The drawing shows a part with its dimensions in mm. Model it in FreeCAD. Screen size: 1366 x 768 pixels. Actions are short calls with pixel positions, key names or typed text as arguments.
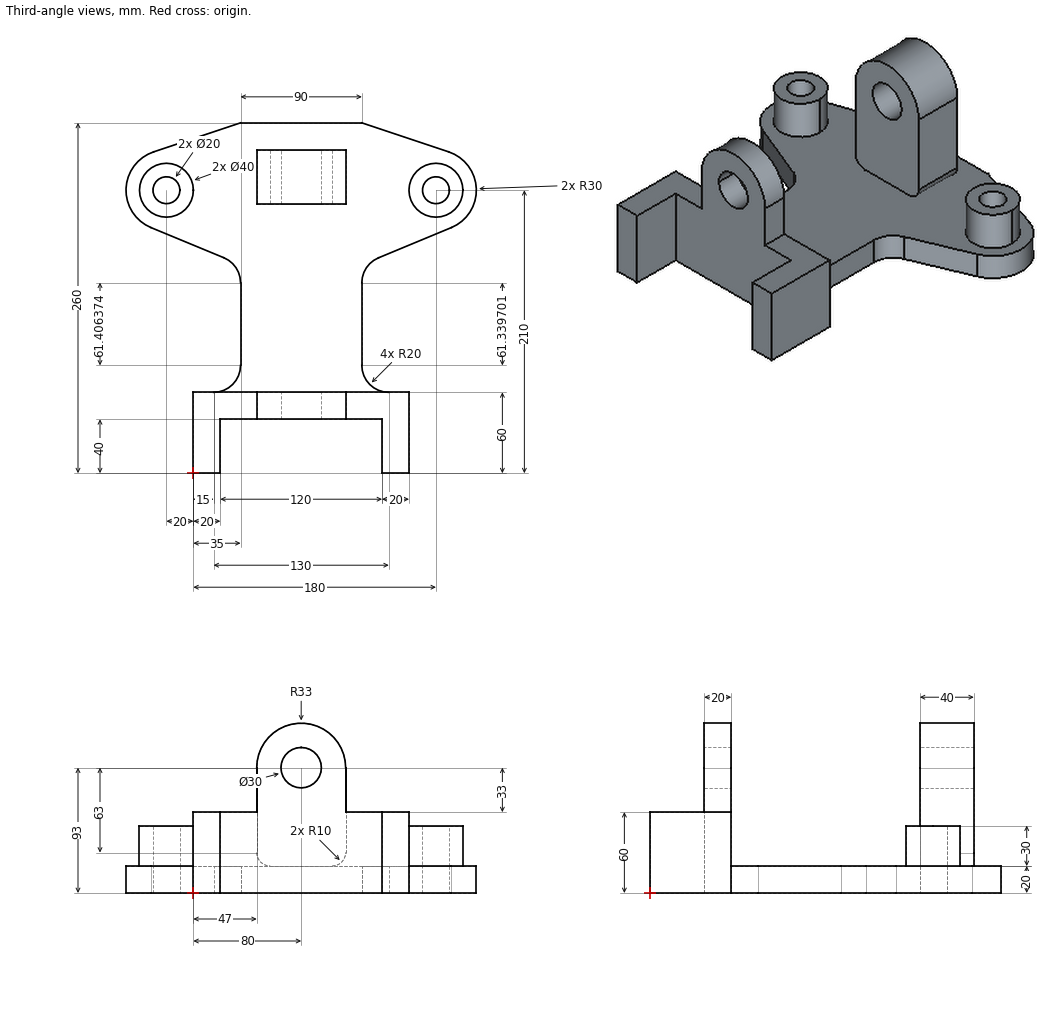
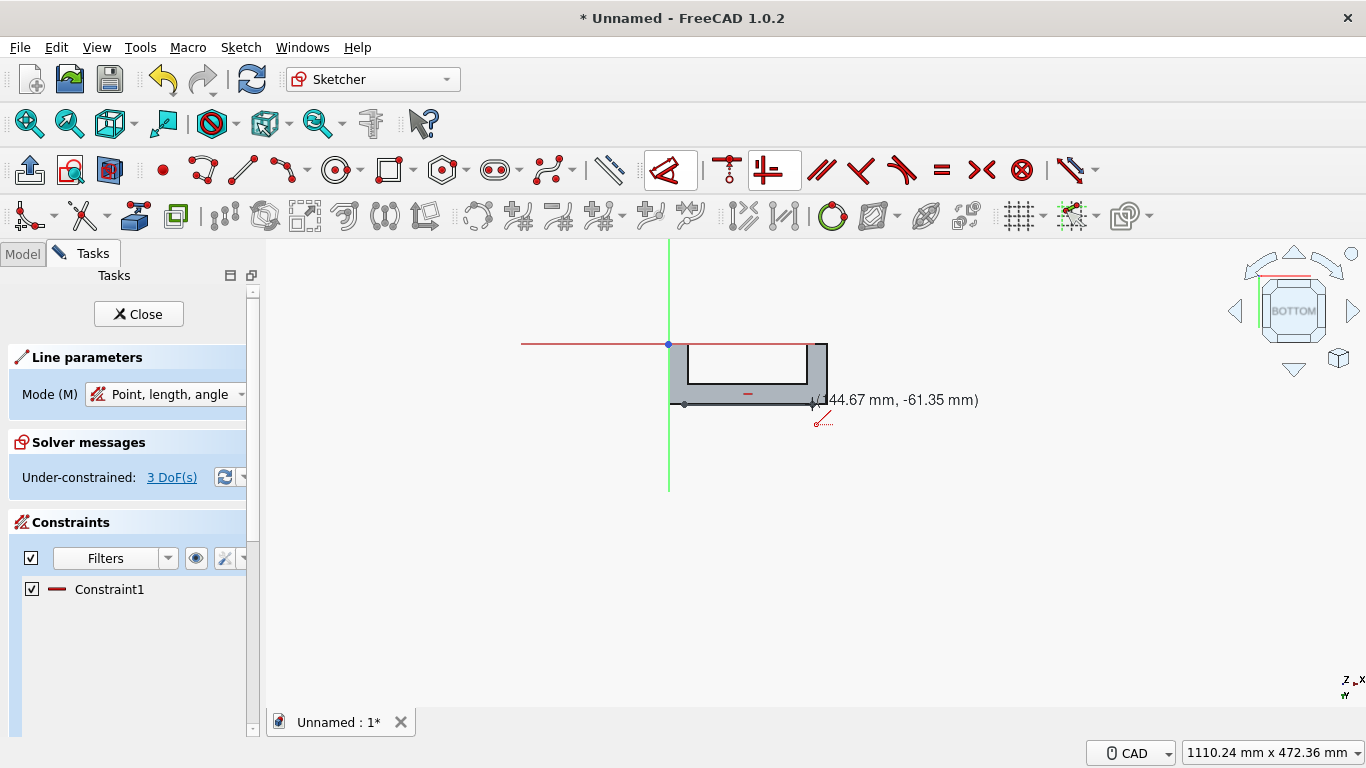
click(793, 423)
click(793, 484)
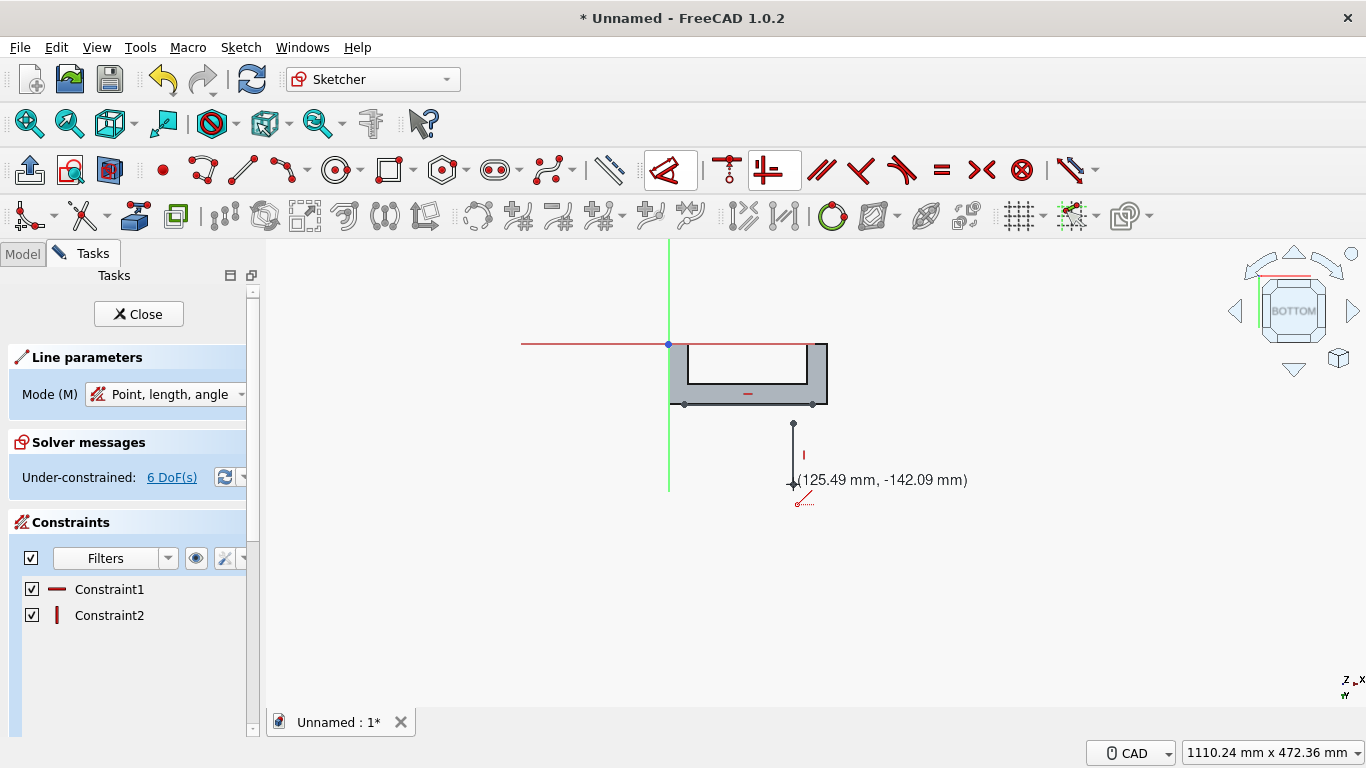
click(805, 503)
click(858, 525)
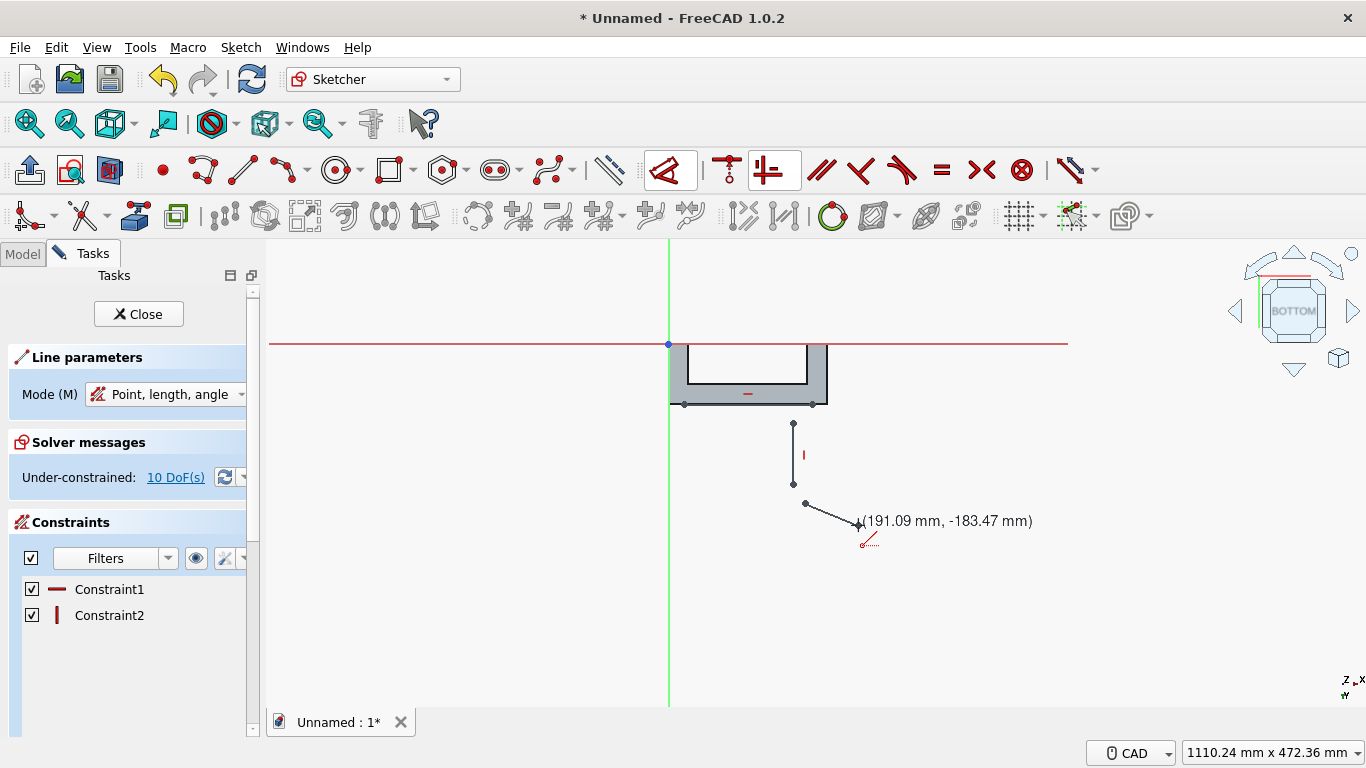
key(g)
key(m)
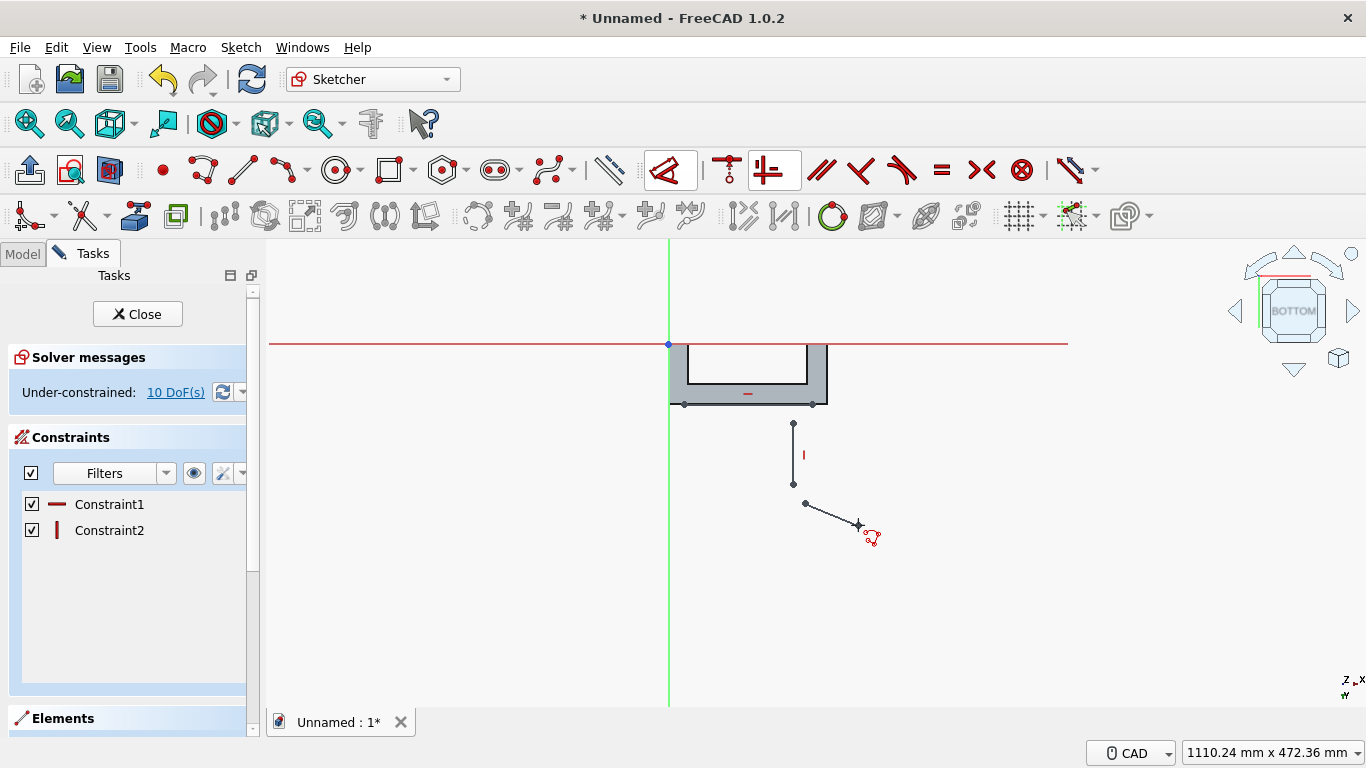
click(856, 580)
click(793, 602)
click(703, 602)
click(639, 580)
right_click(639, 580)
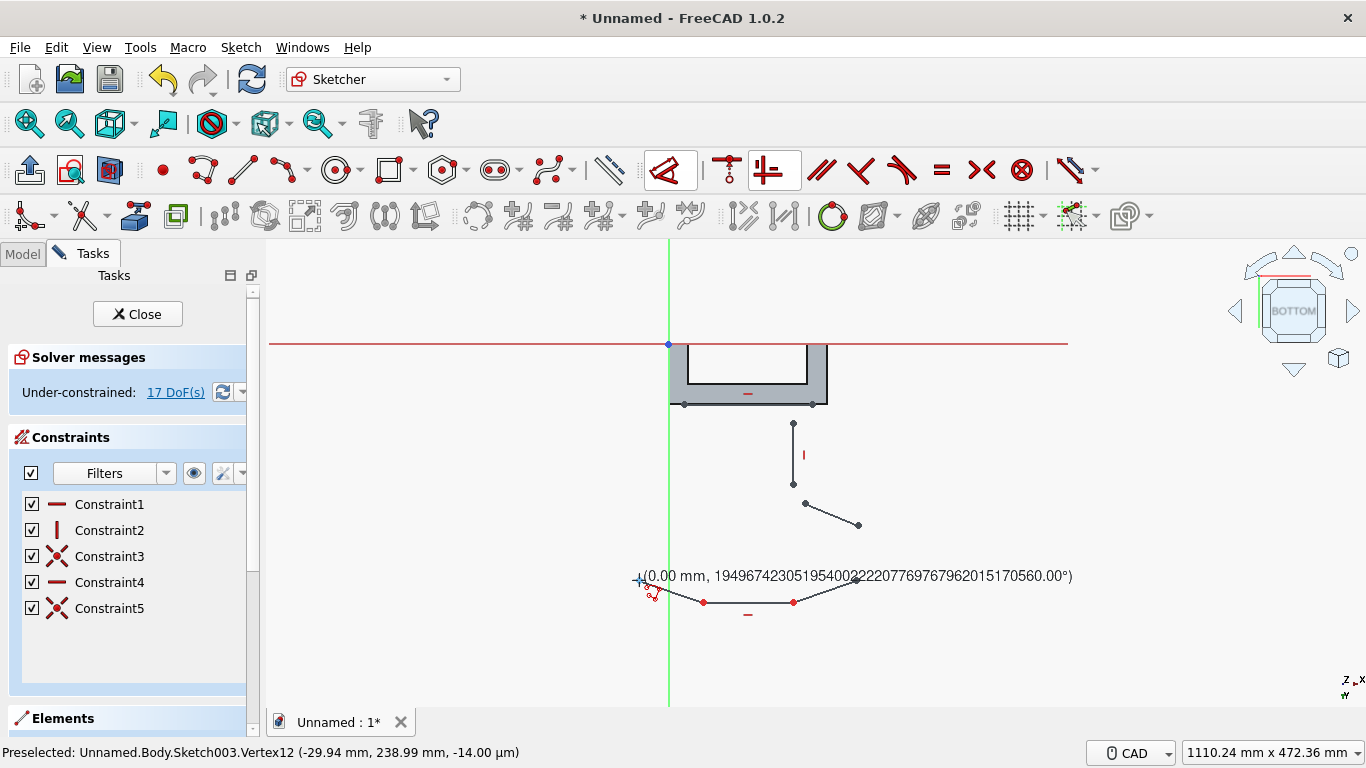
click(244, 170)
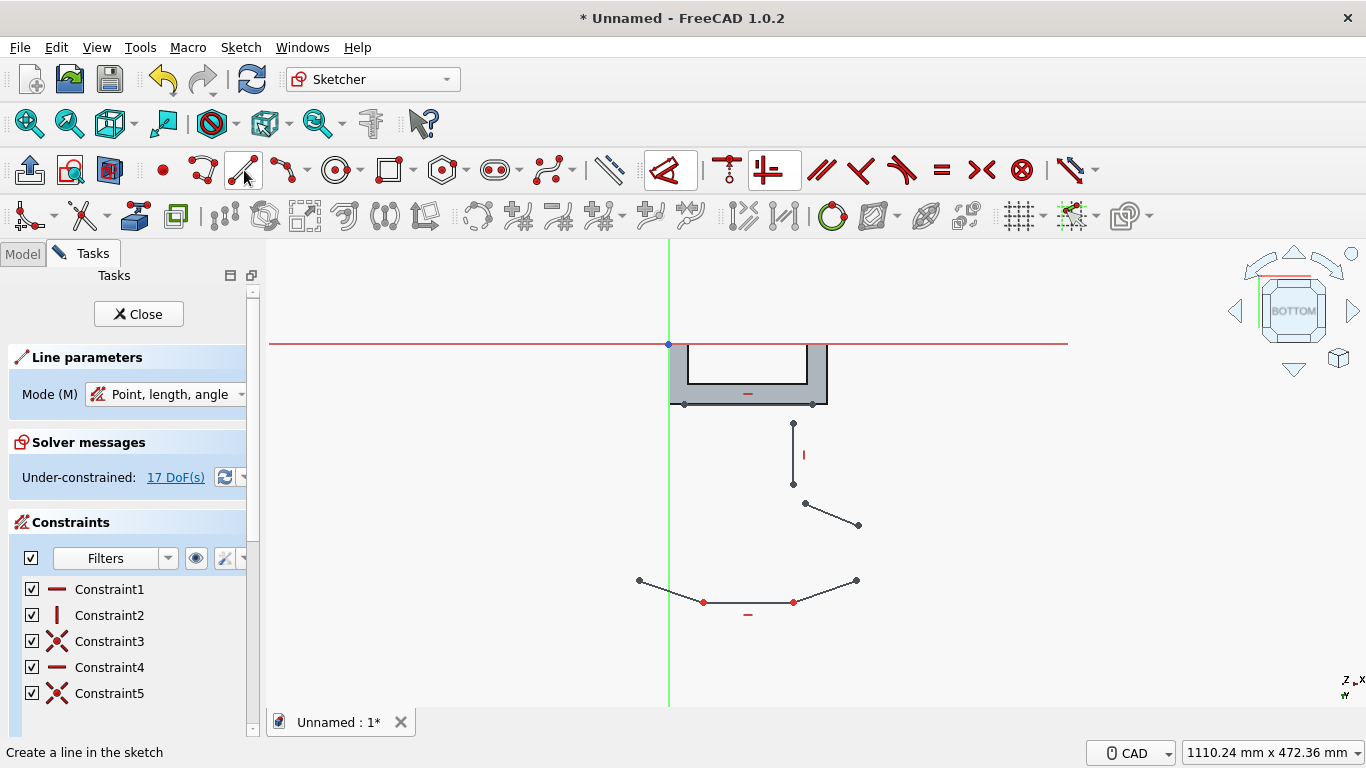
click(637, 525)
click(691, 503)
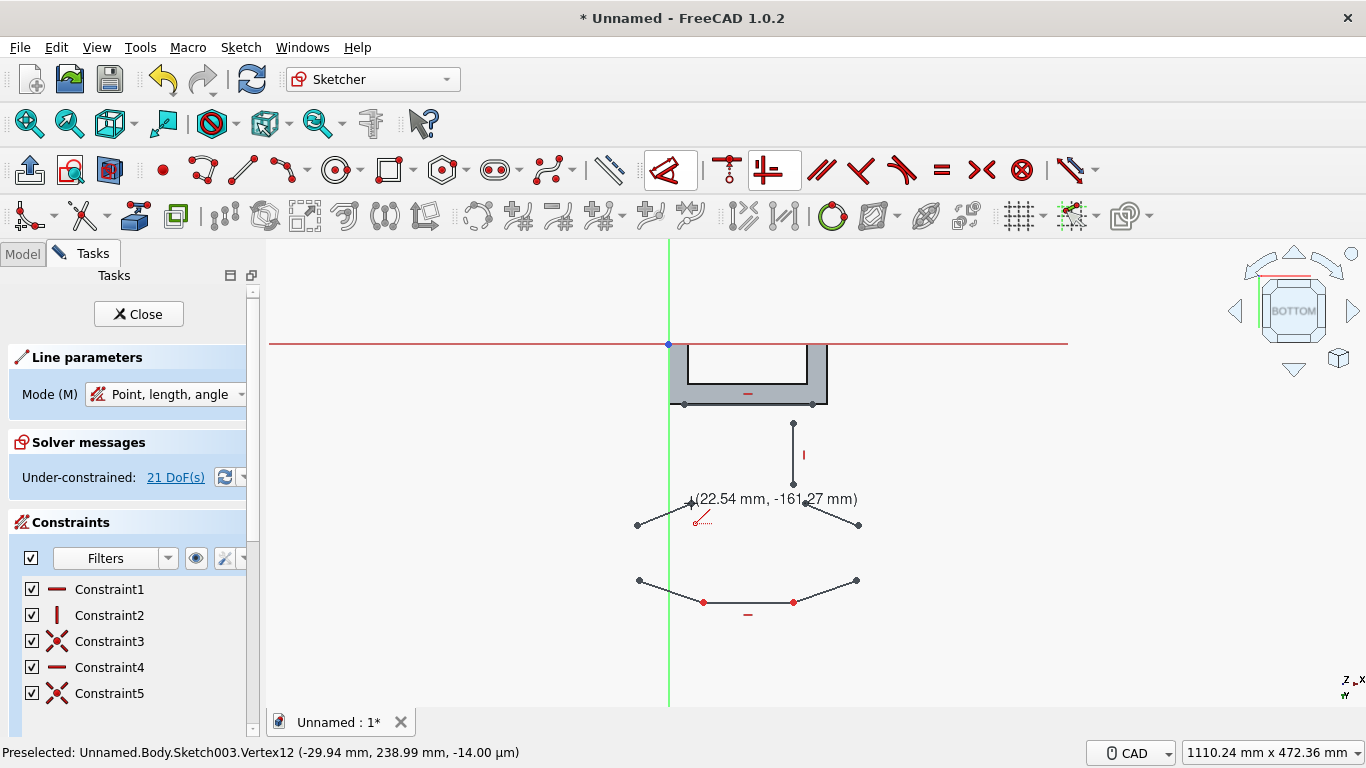
click(703, 484)
click(703, 423)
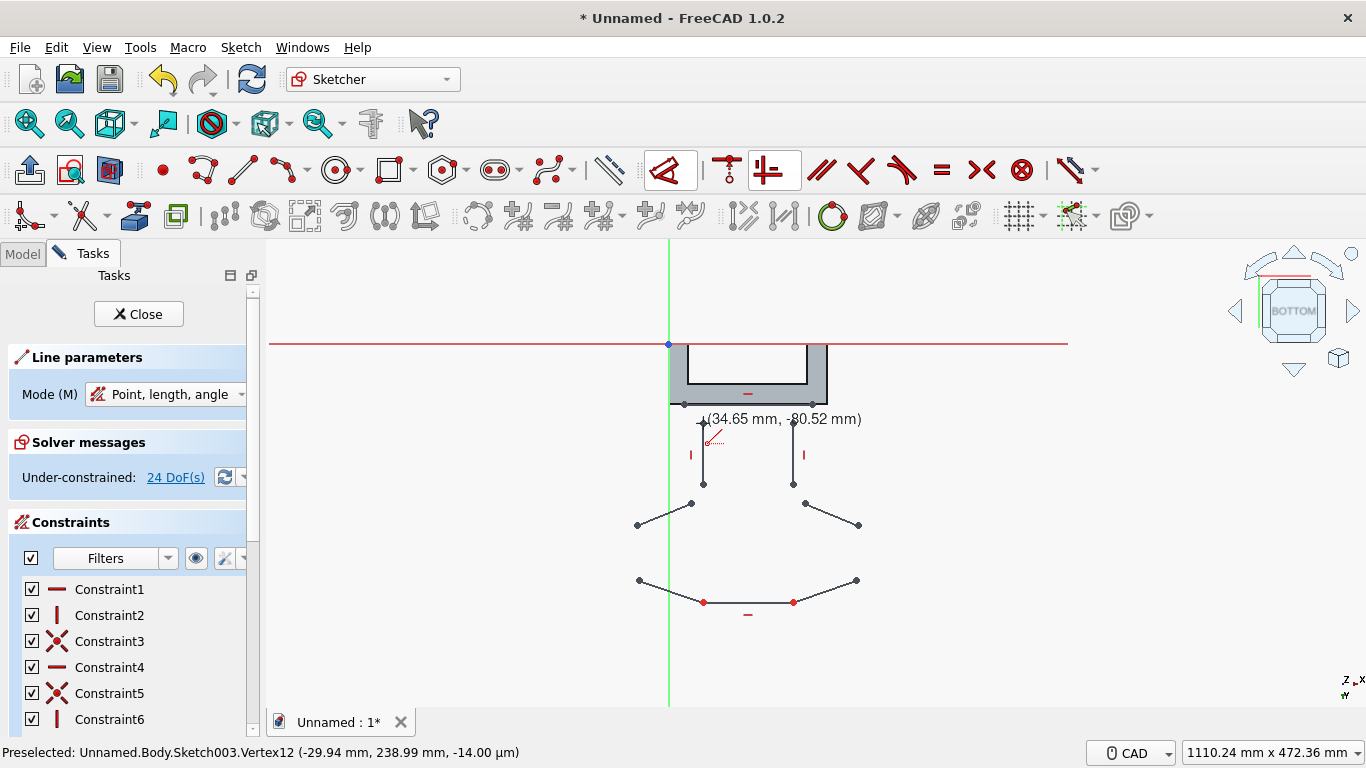
click(284, 170)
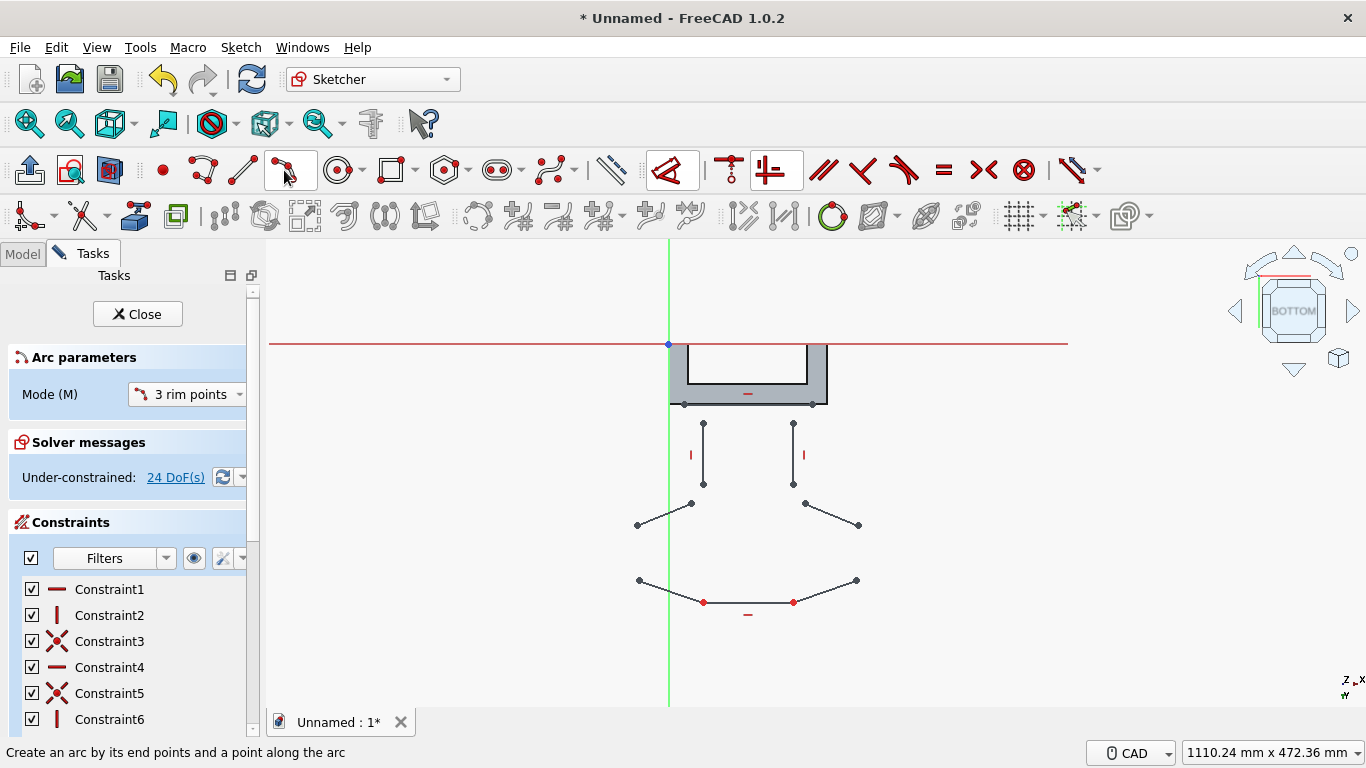
click(812, 405)
click(793, 424)